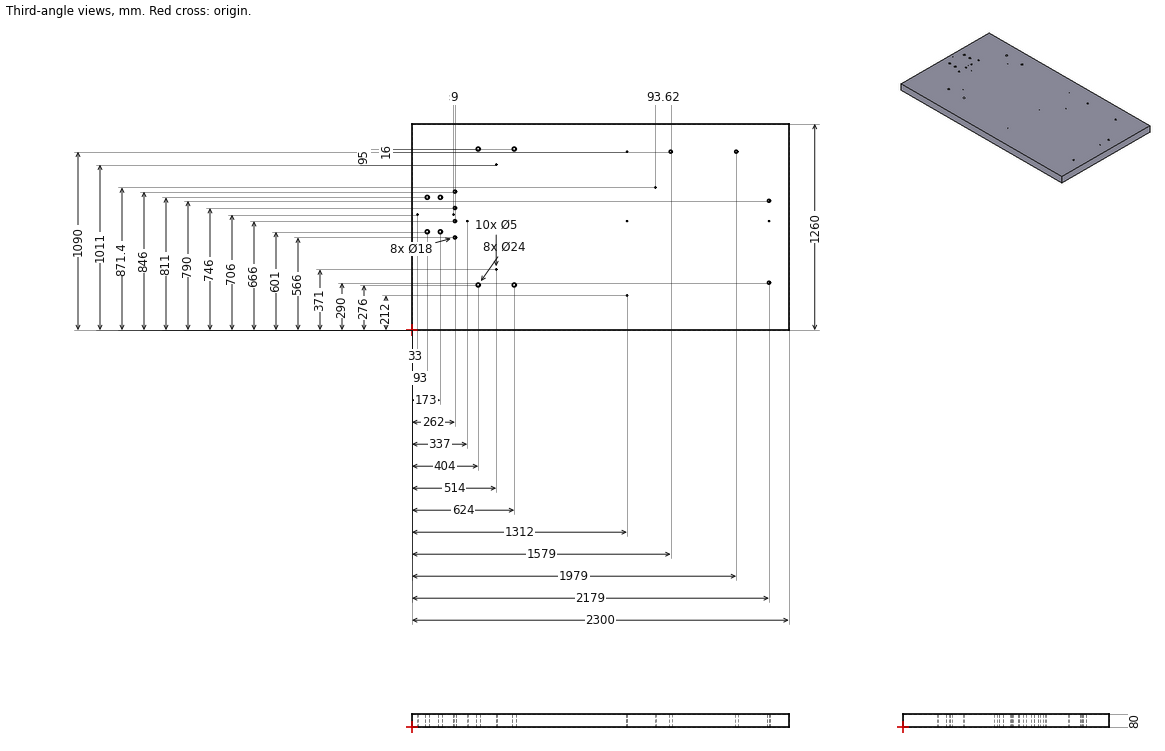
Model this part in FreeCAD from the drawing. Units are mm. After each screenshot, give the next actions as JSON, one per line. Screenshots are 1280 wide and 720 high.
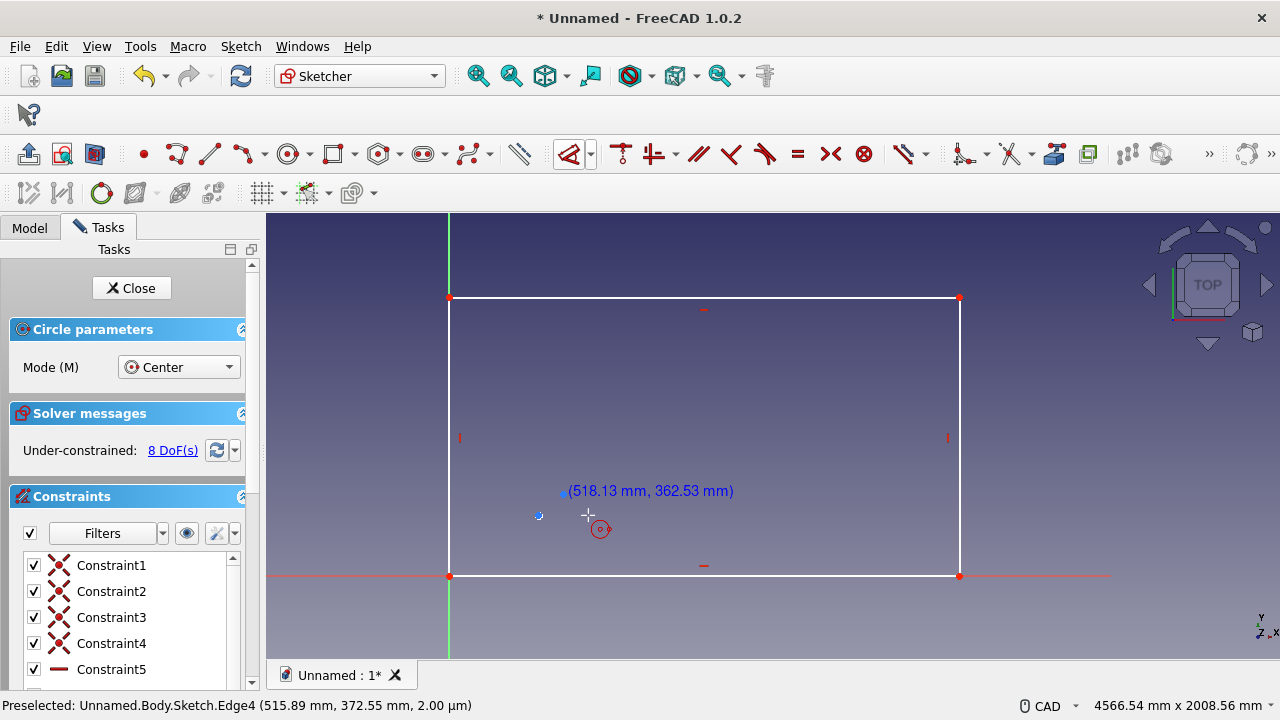
{"action": "left_click", "coordinate": [588, 515]}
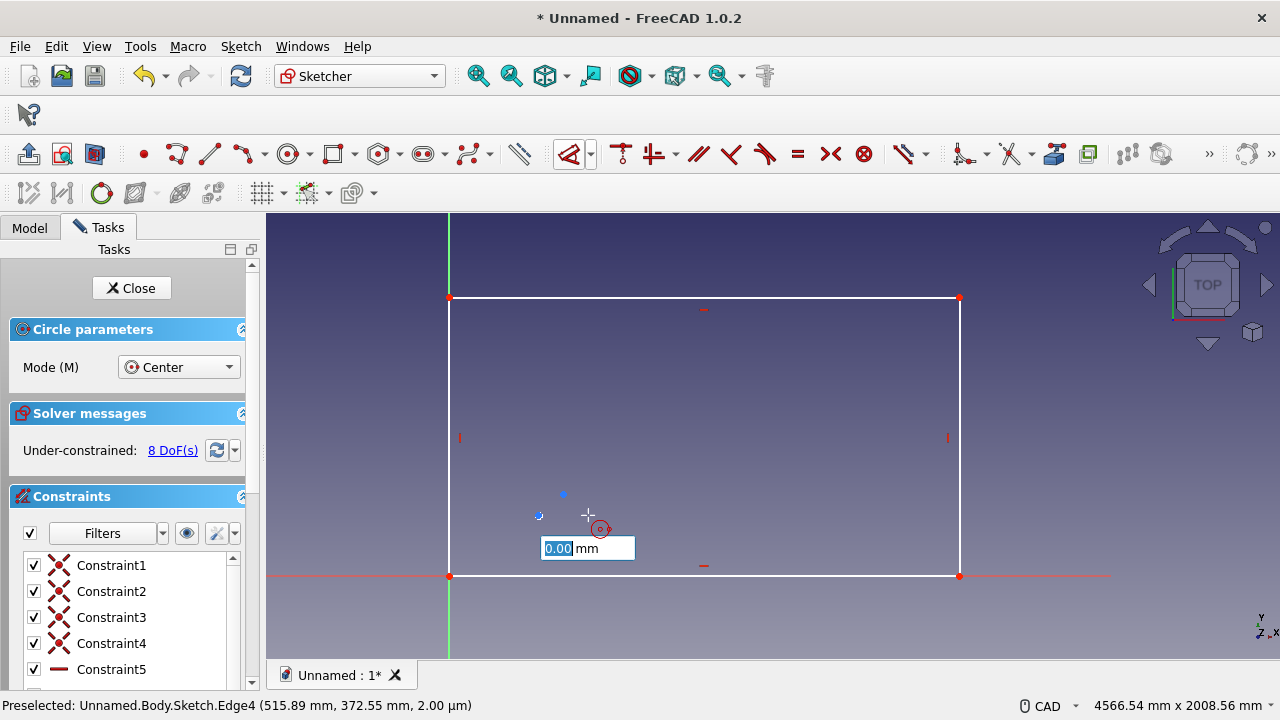
{"action": "scroll", "coordinate": [589, 513], "scroll_direction": "up", "scroll_amount": 9}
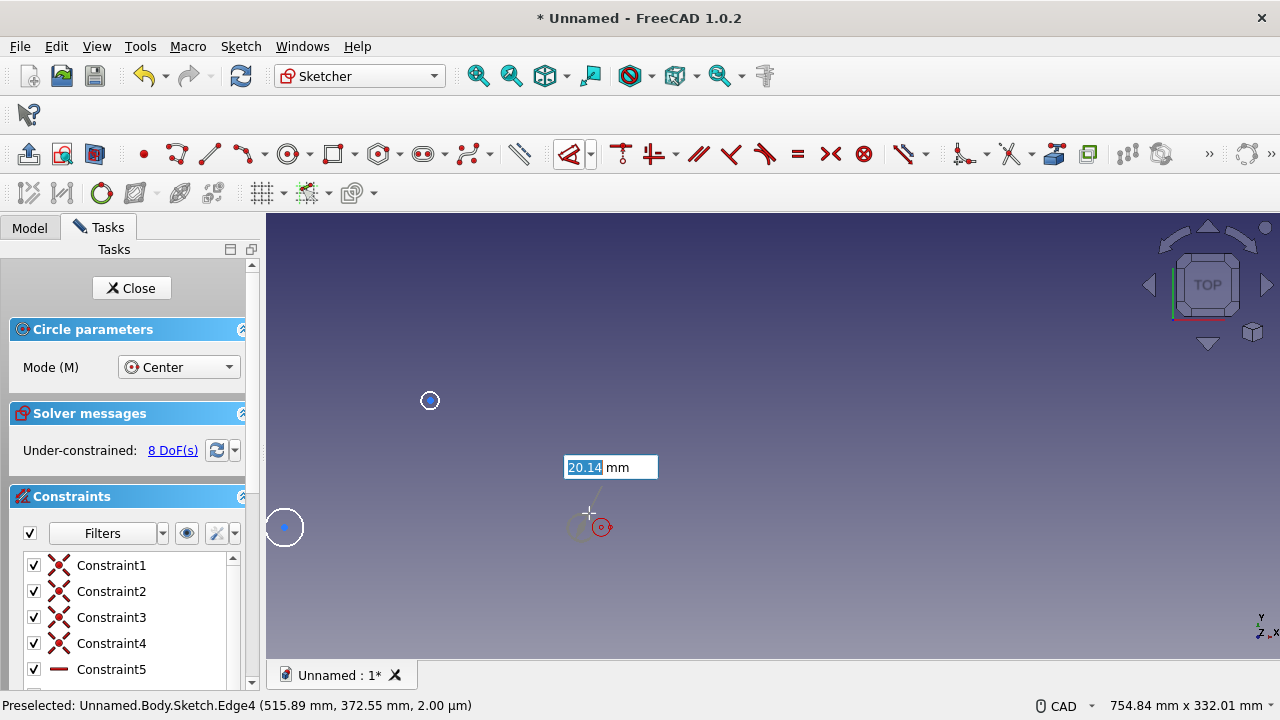
{"action": "left_click", "coordinate": [590, 511]}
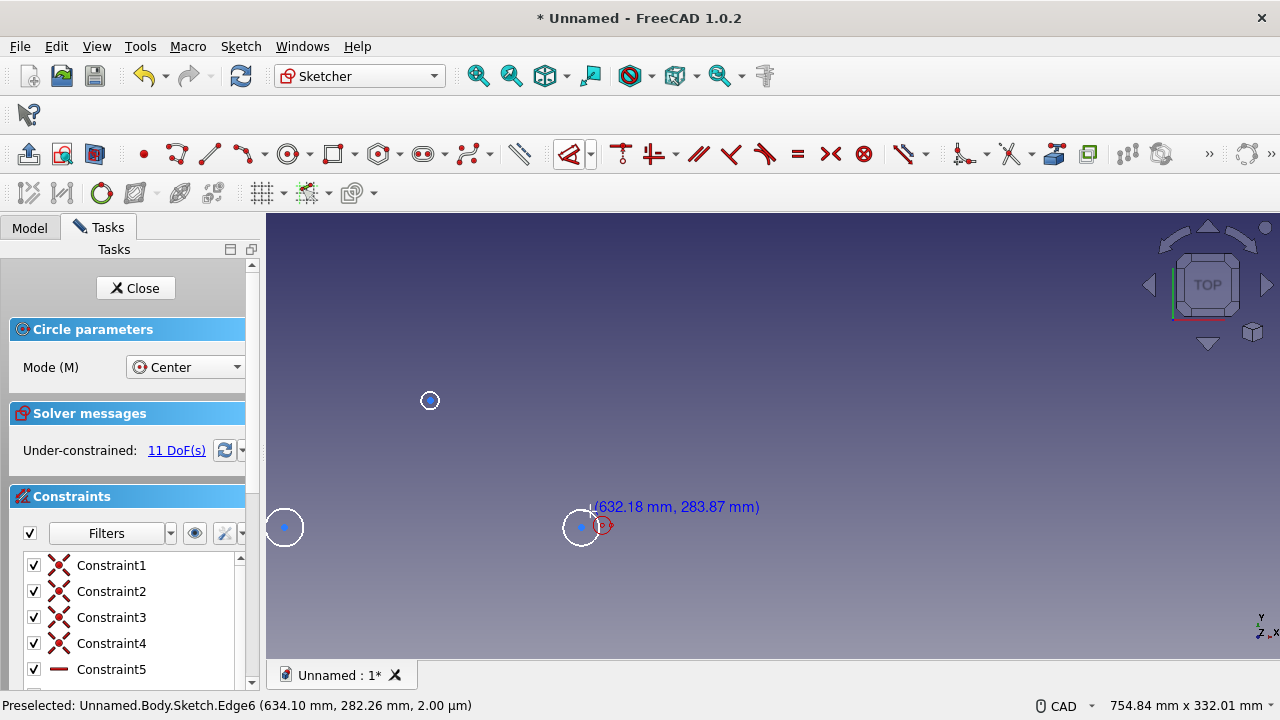
{"action": "scroll", "coordinate": [589, 513], "scroll_direction": "down", "scroll_amount": 9}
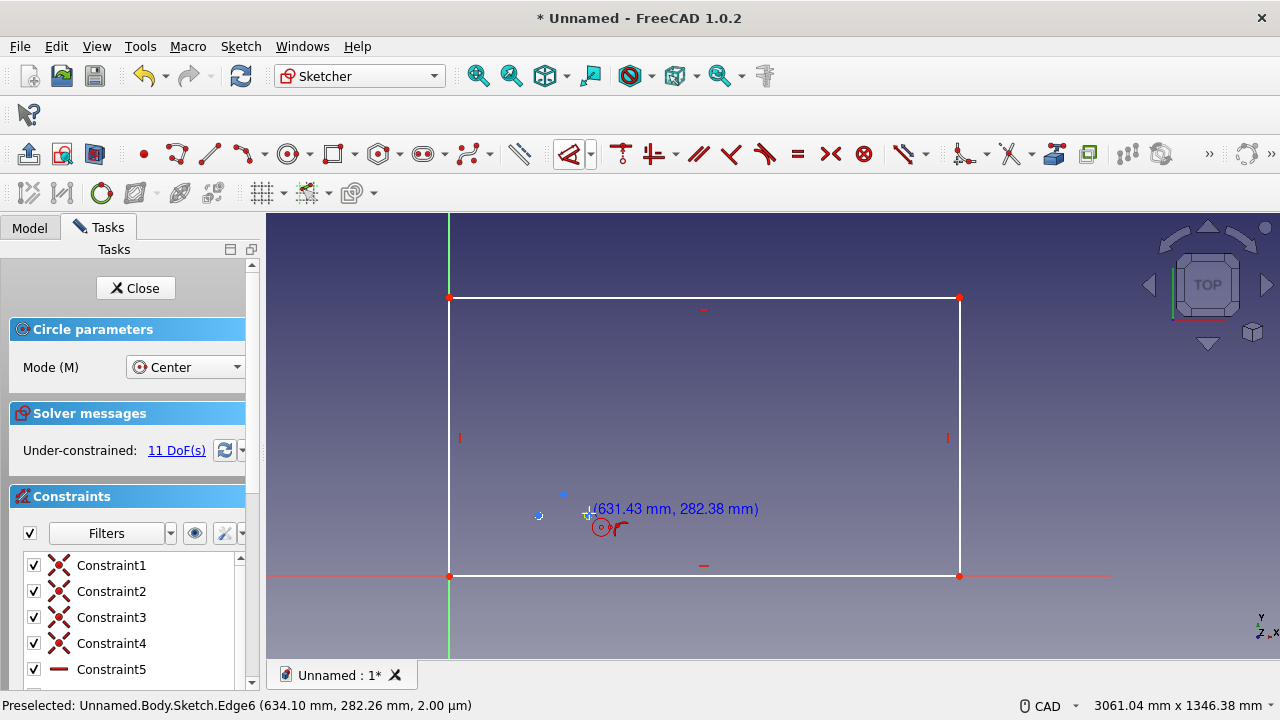
{"action": "scroll", "coordinate": [470, 443], "scroll_direction": "up", "scroll_amount": 11}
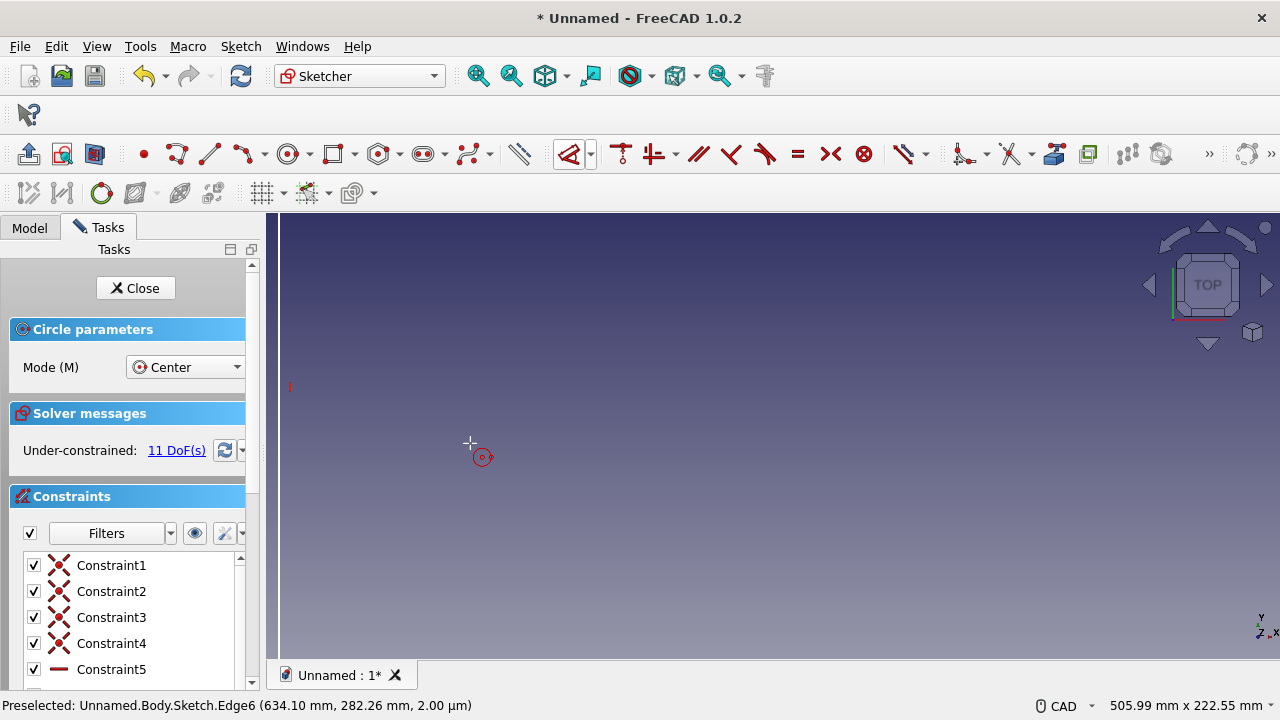
{"action": "scroll", "coordinate": [470, 443], "scroll_direction": "down", "scroll_amount": 11}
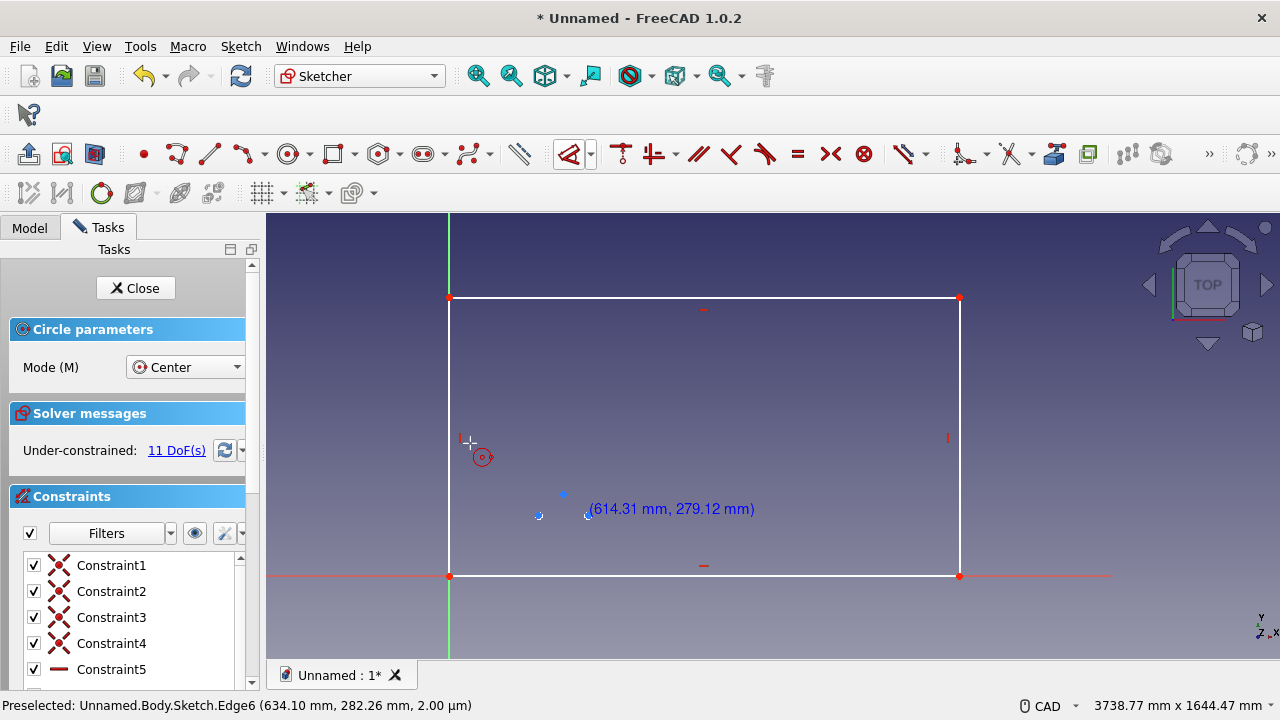
{"action": "left_click", "coordinate": [470, 443]}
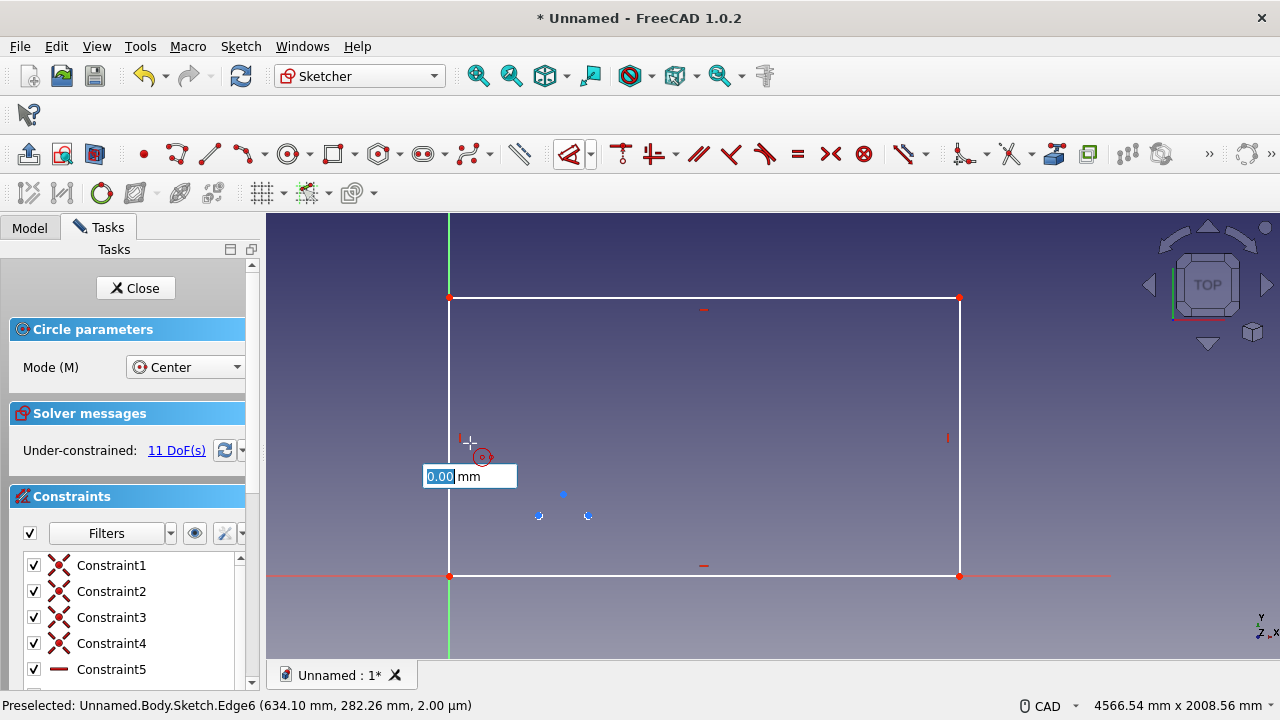
{"action": "scroll", "coordinate": [472, 441], "scroll_direction": "up", "scroll_amount": 9}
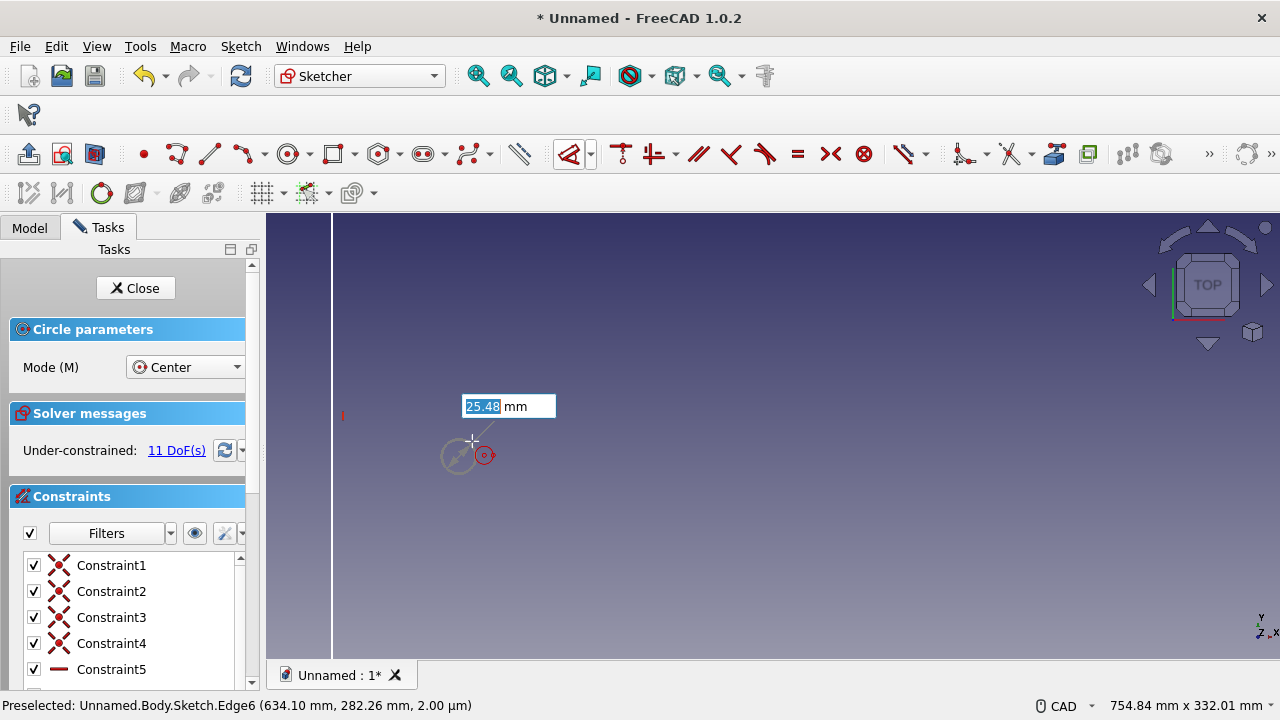
{"action": "left_click", "coordinate": [468, 439]}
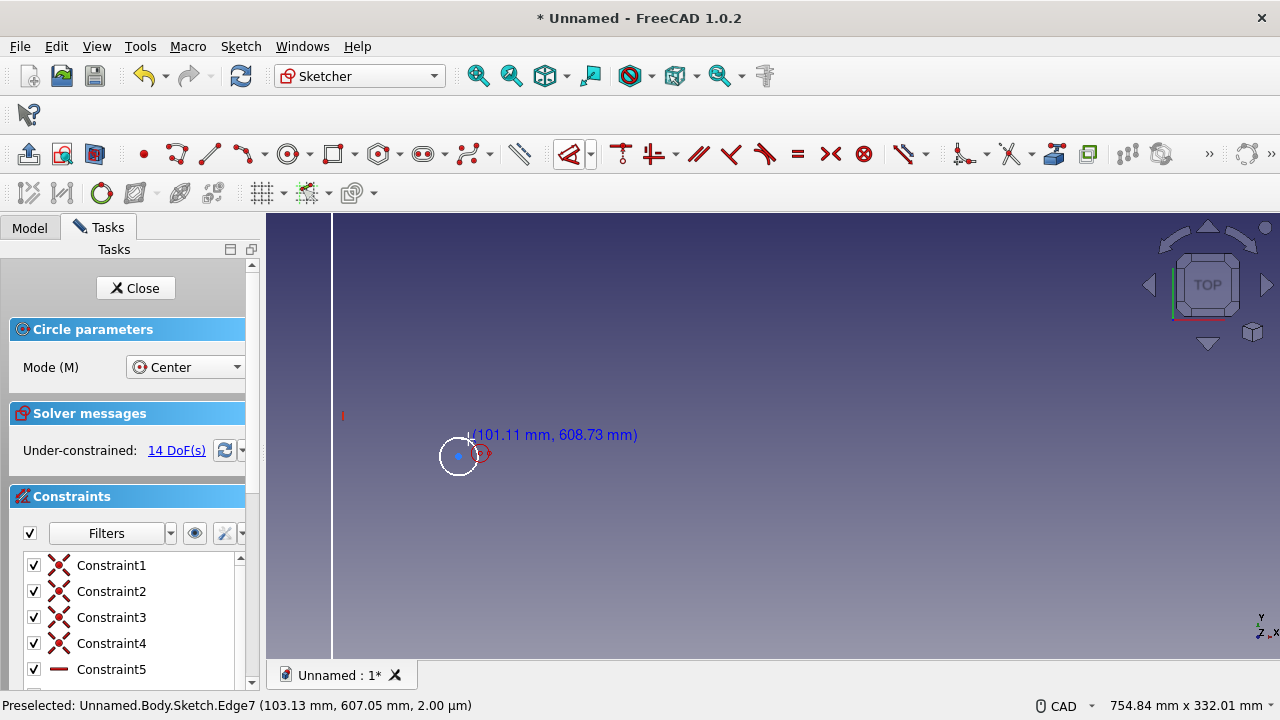
{"action": "scroll", "coordinate": [684, 497], "scroll_direction": "up", "scroll_amount": 4}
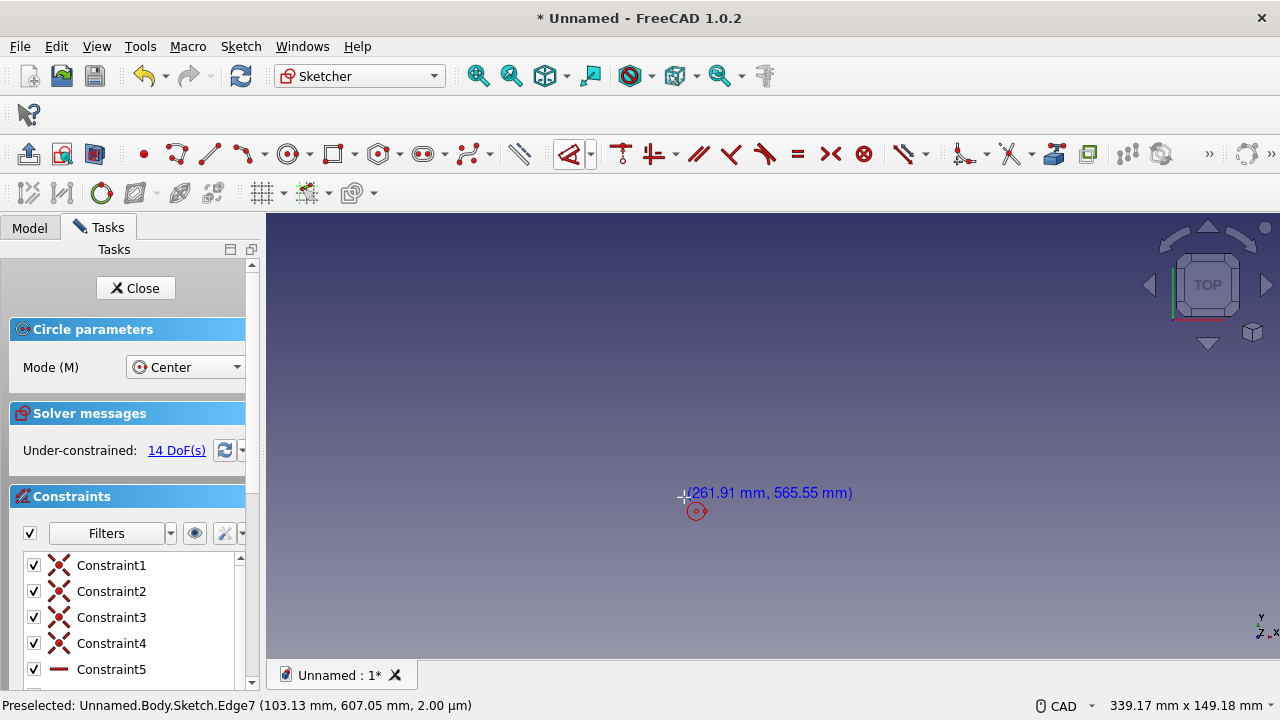
{"action": "scroll", "coordinate": [493, 446], "scroll_direction": "down", "scroll_amount": 13}